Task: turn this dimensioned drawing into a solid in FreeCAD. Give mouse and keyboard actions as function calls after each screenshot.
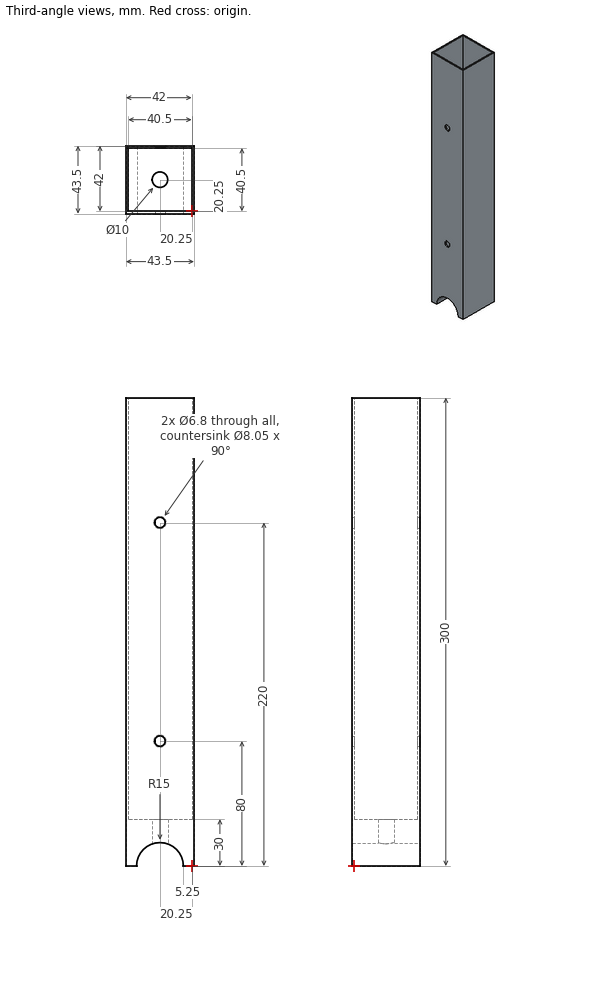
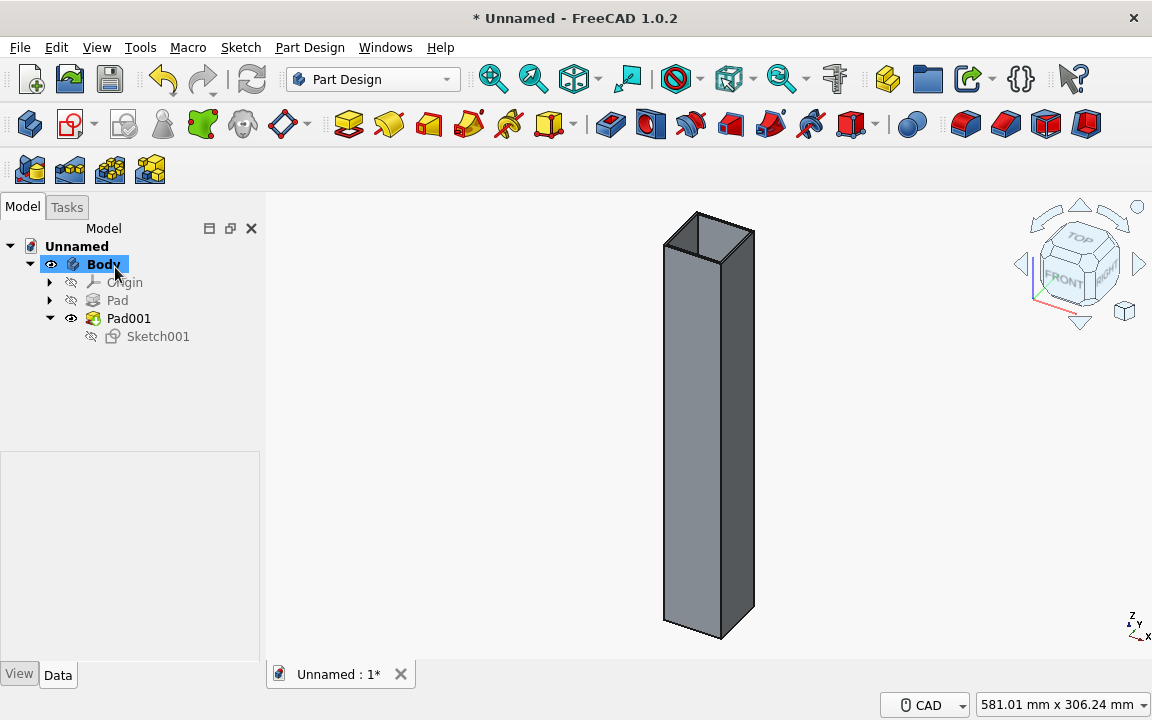
key(4)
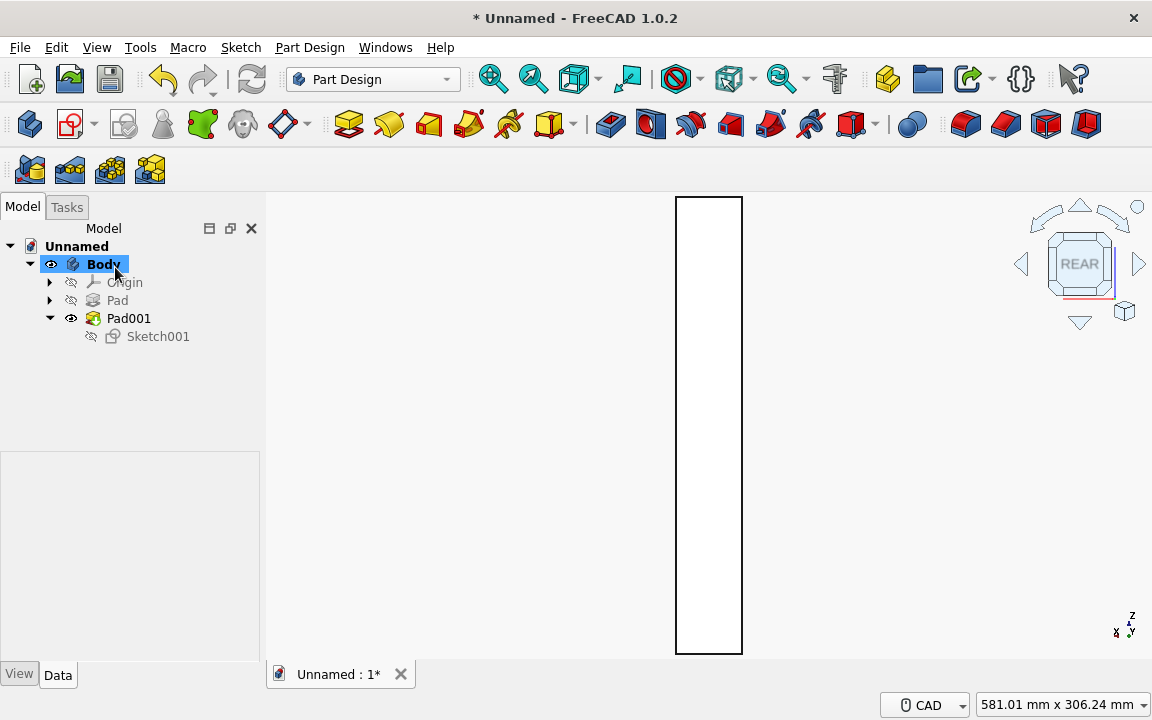
click(709, 294)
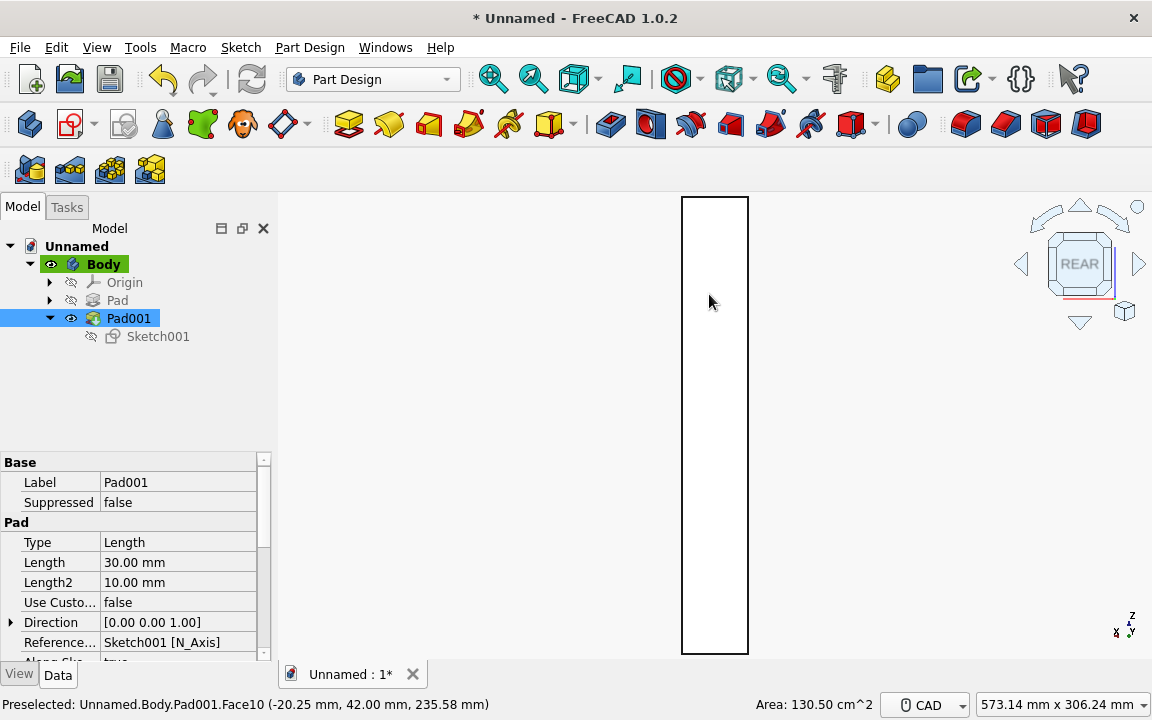
click(70, 124)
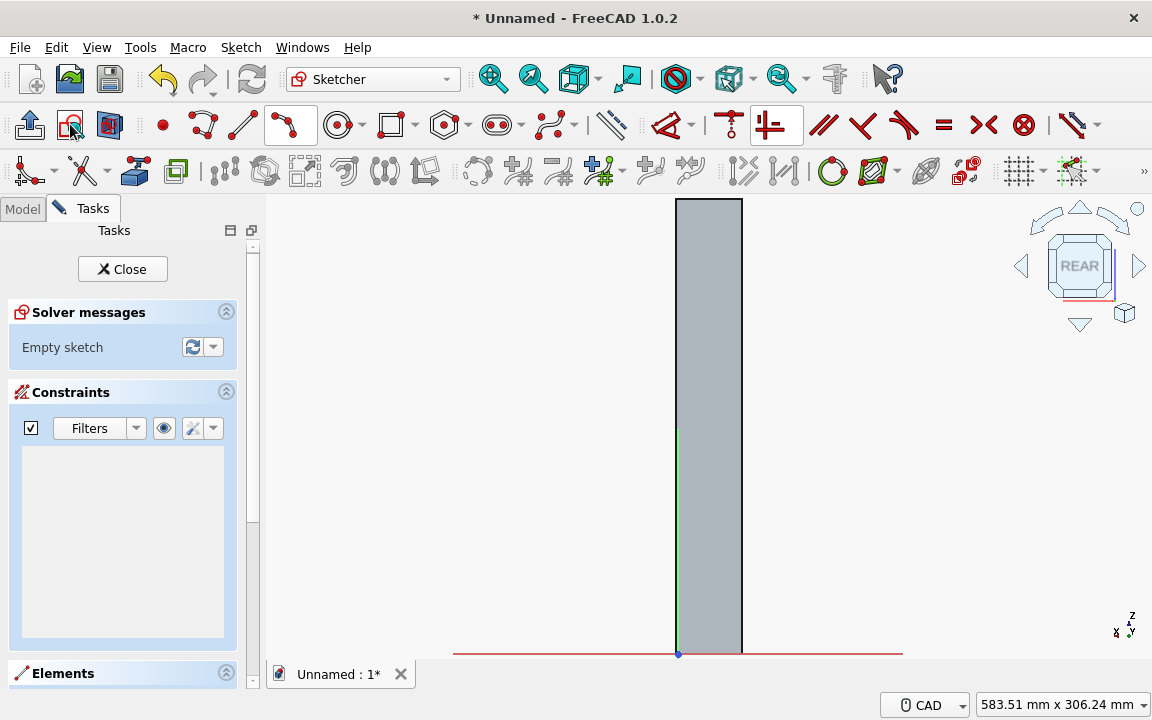
scroll(389, 222, down, 1)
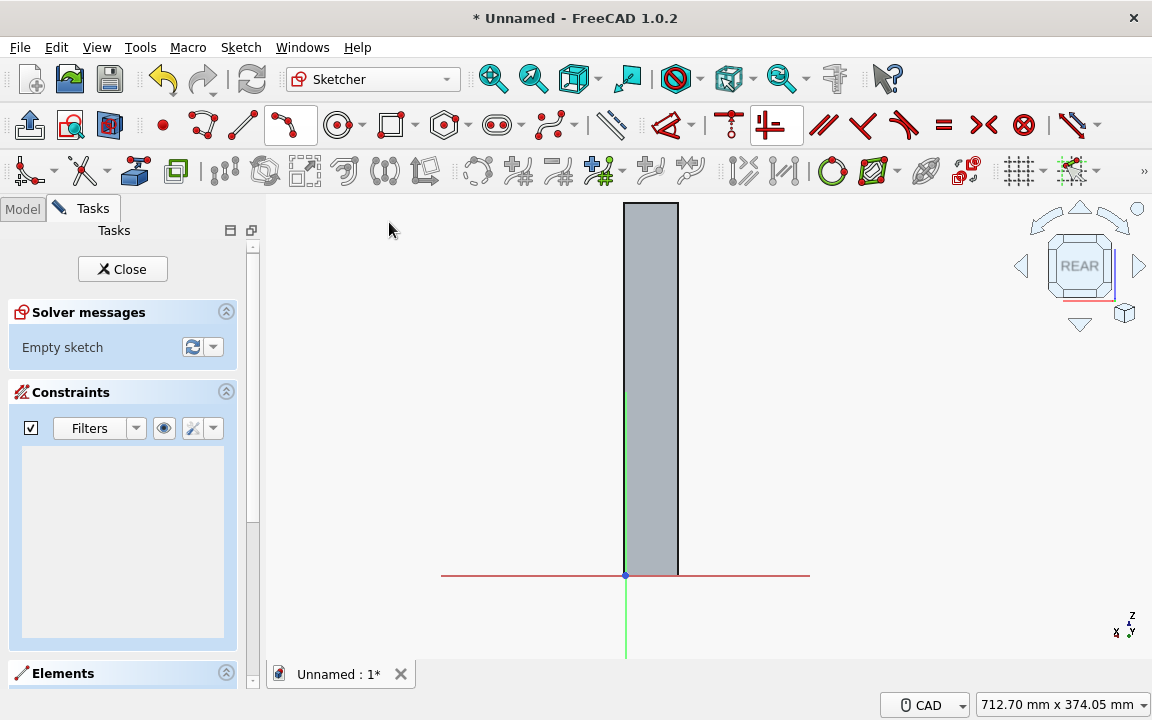
click(338, 126)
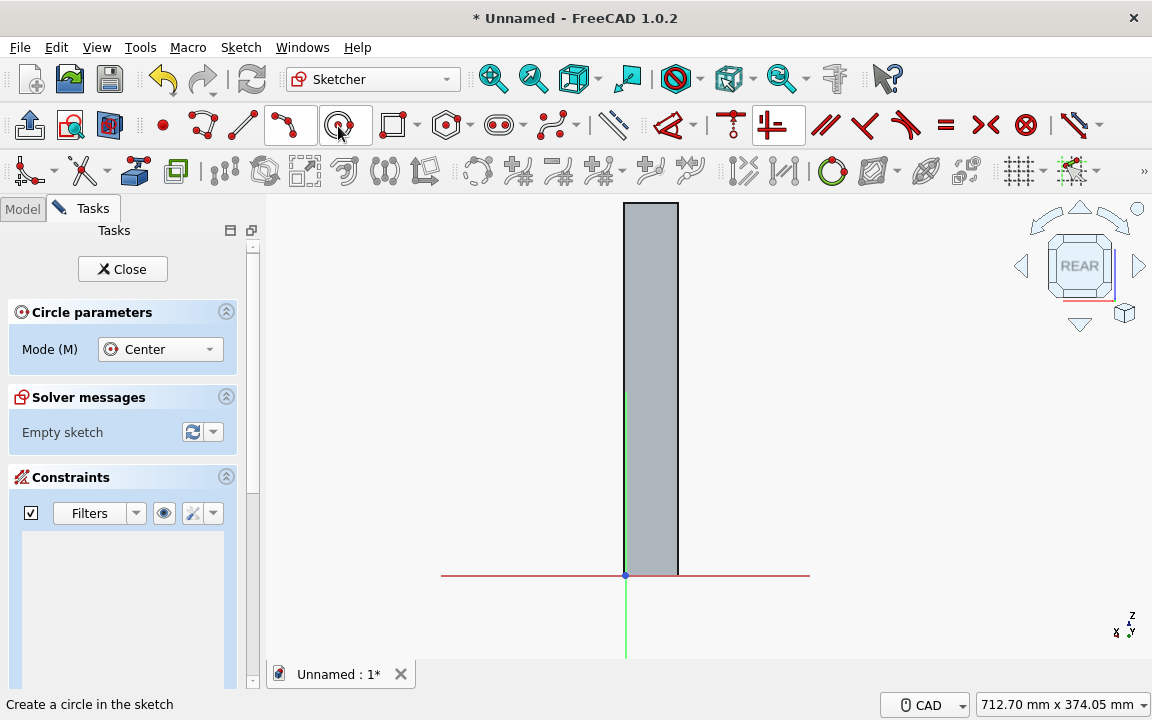
scroll(651, 302, up, 9)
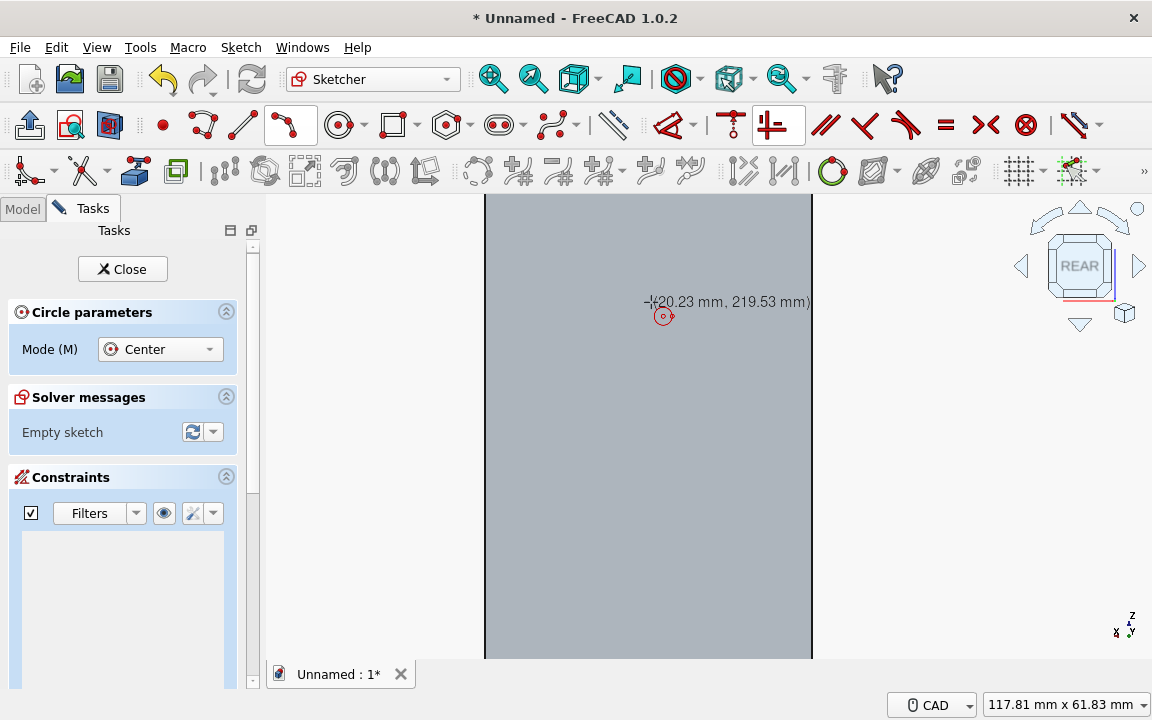
scroll(651, 290, down, 9)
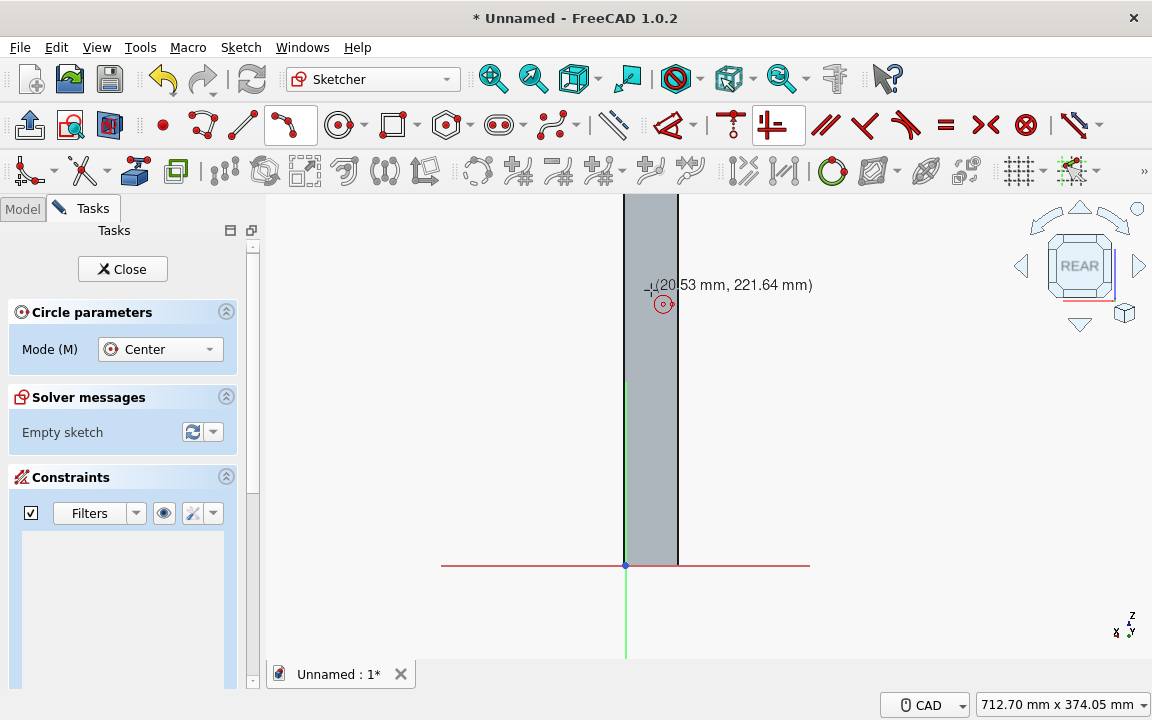
click(651, 292)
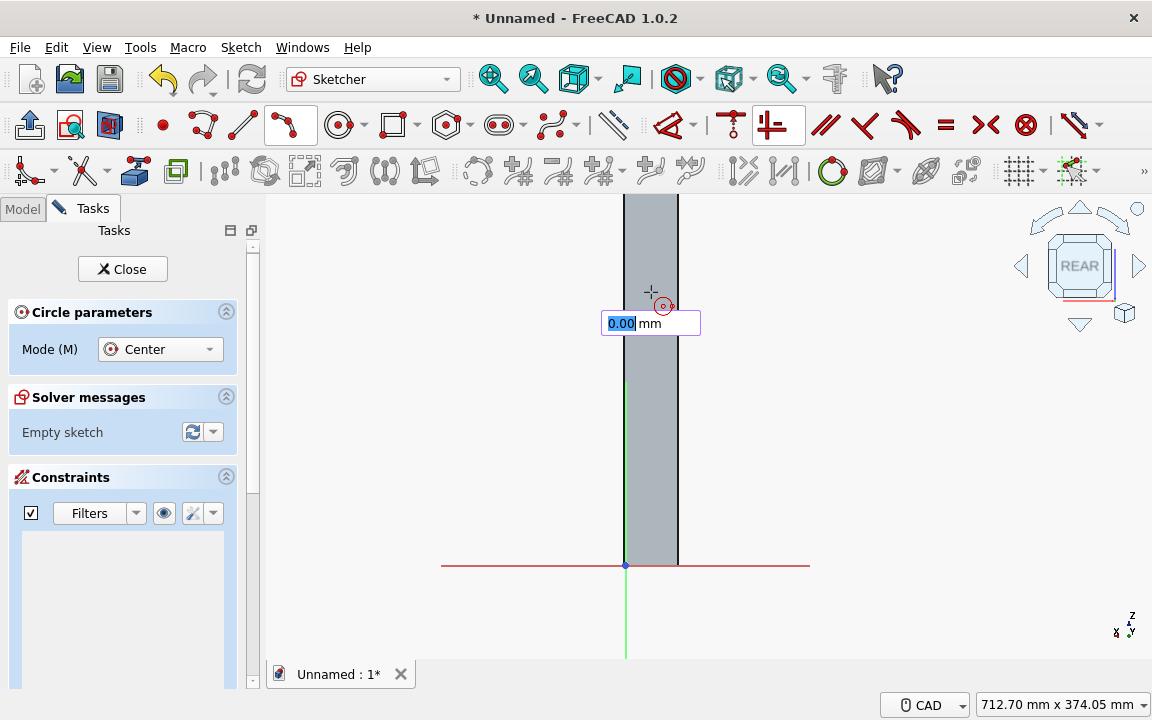
scroll(654, 289, up, 7)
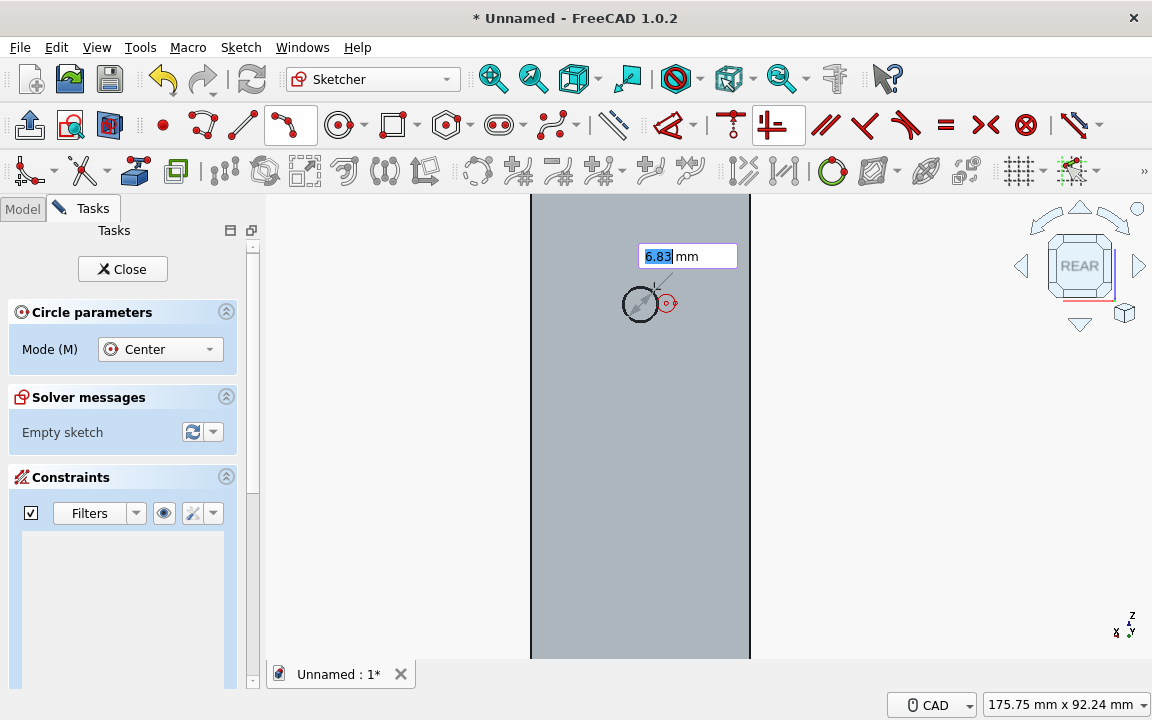
click(653, 290)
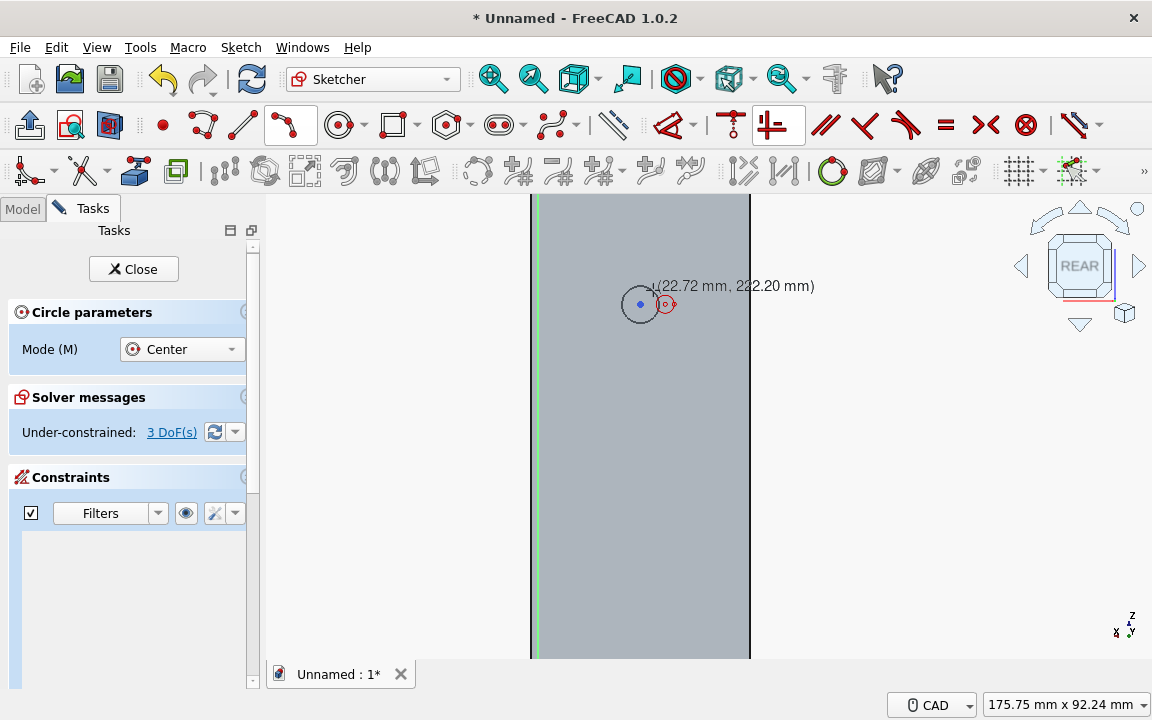
scroll(654, 289, down, 7)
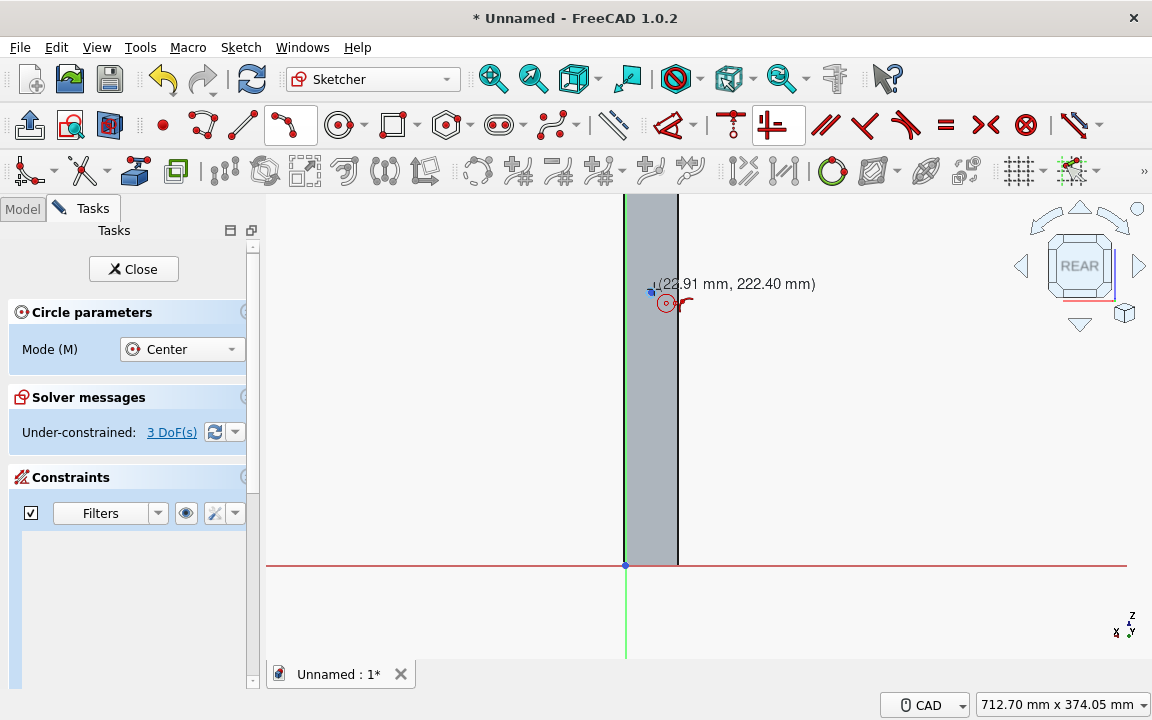
scroll(651, 466, up, 9)